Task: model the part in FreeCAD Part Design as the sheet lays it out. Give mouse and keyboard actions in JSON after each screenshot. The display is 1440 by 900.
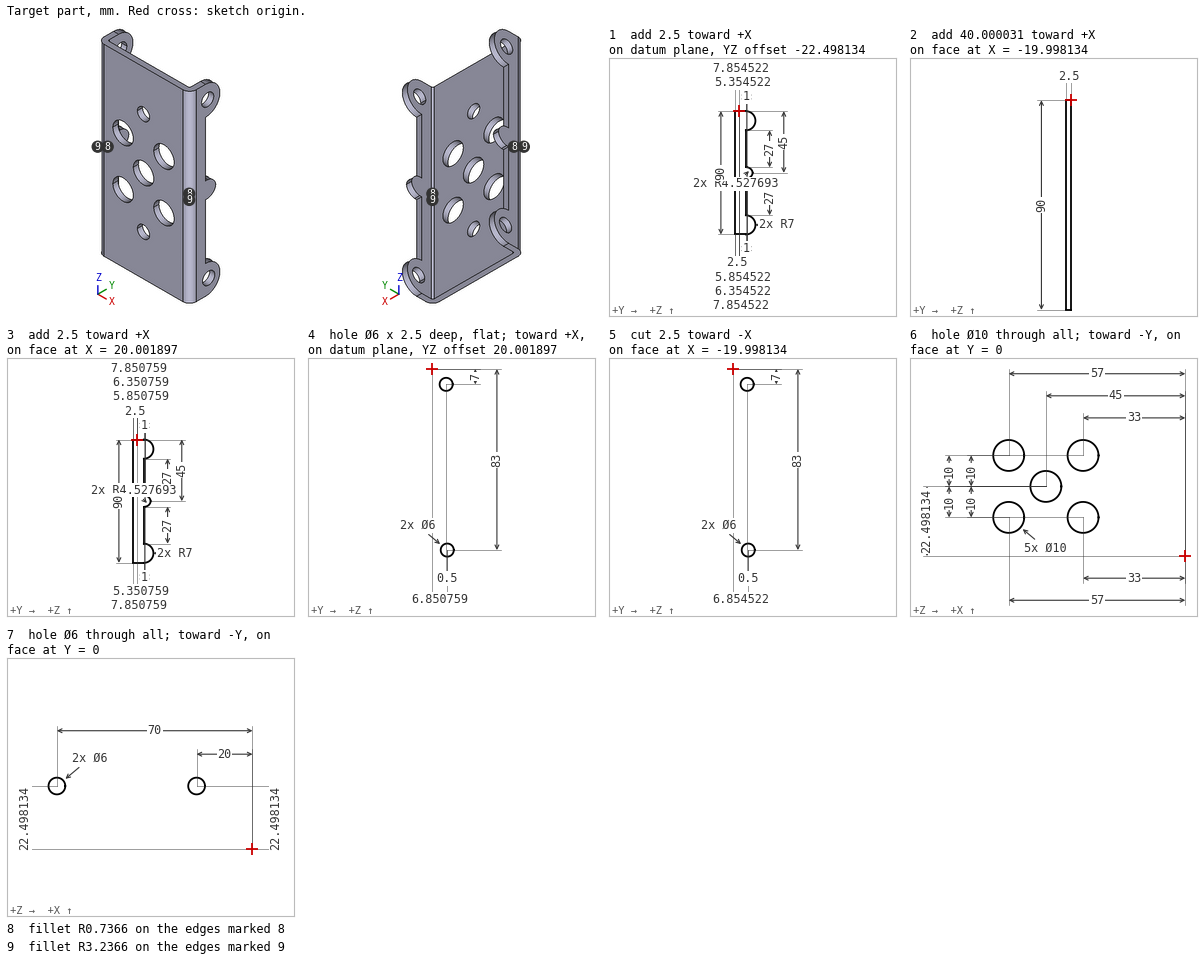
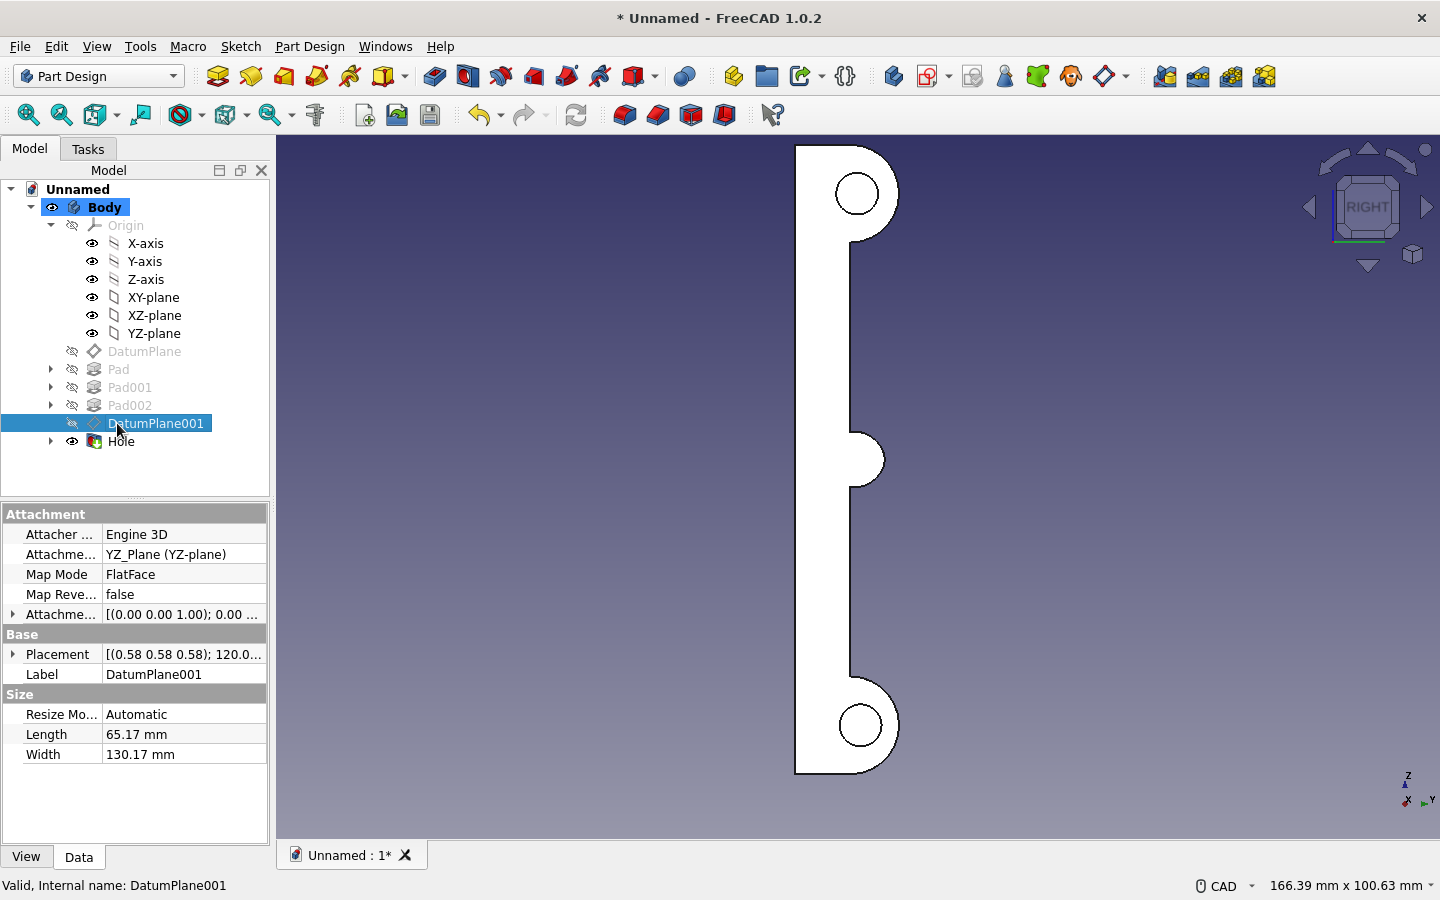
{"action": "left_click", "coordinate": [856, 728]}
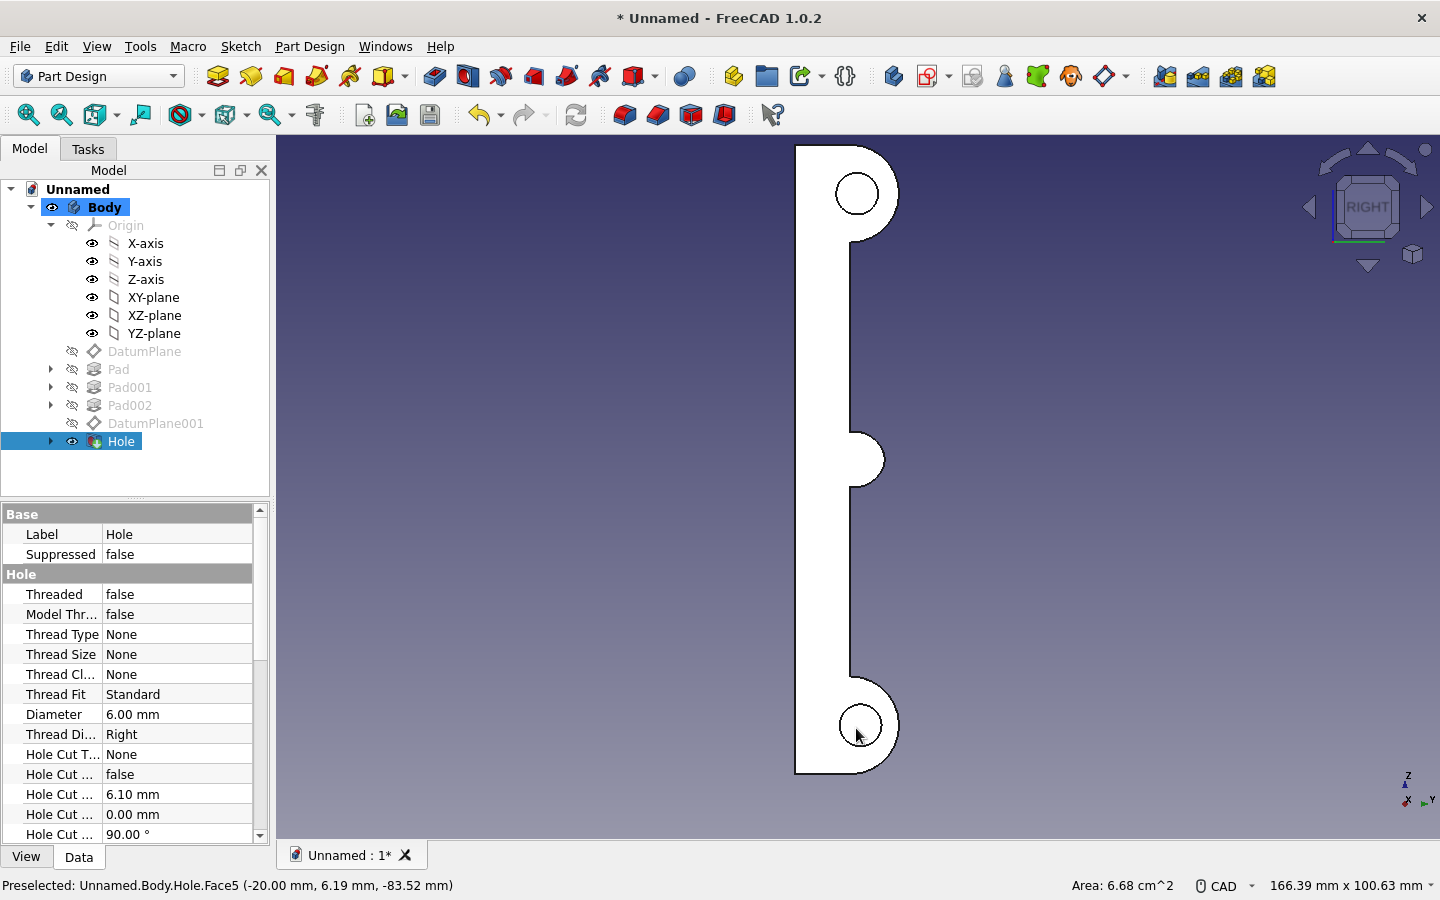
{"action": "left_click", "coordinate": [926, 76]}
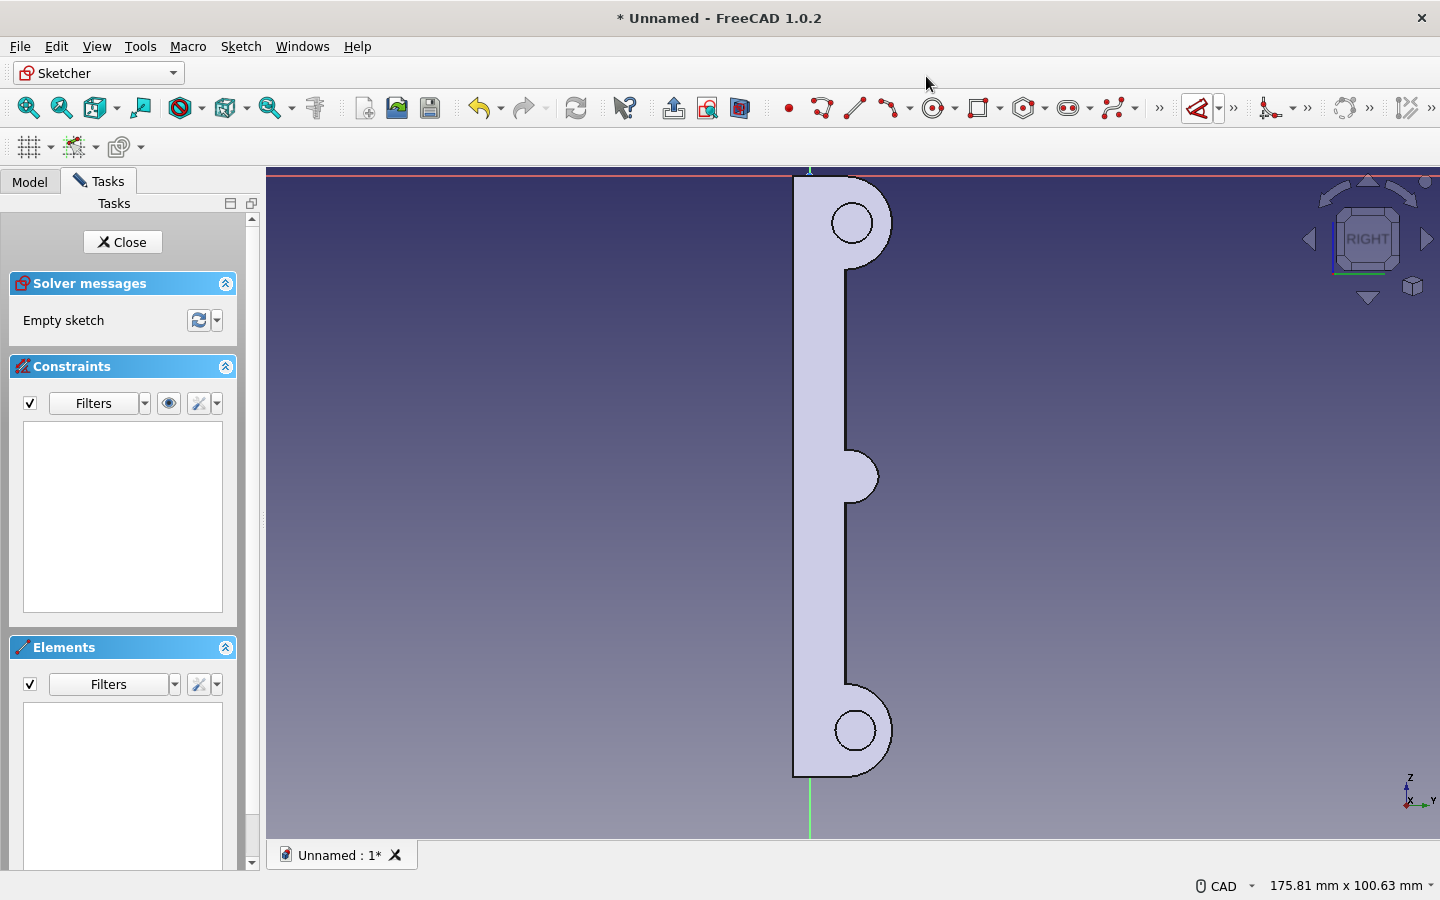
{"action": "key", "text": "q s"}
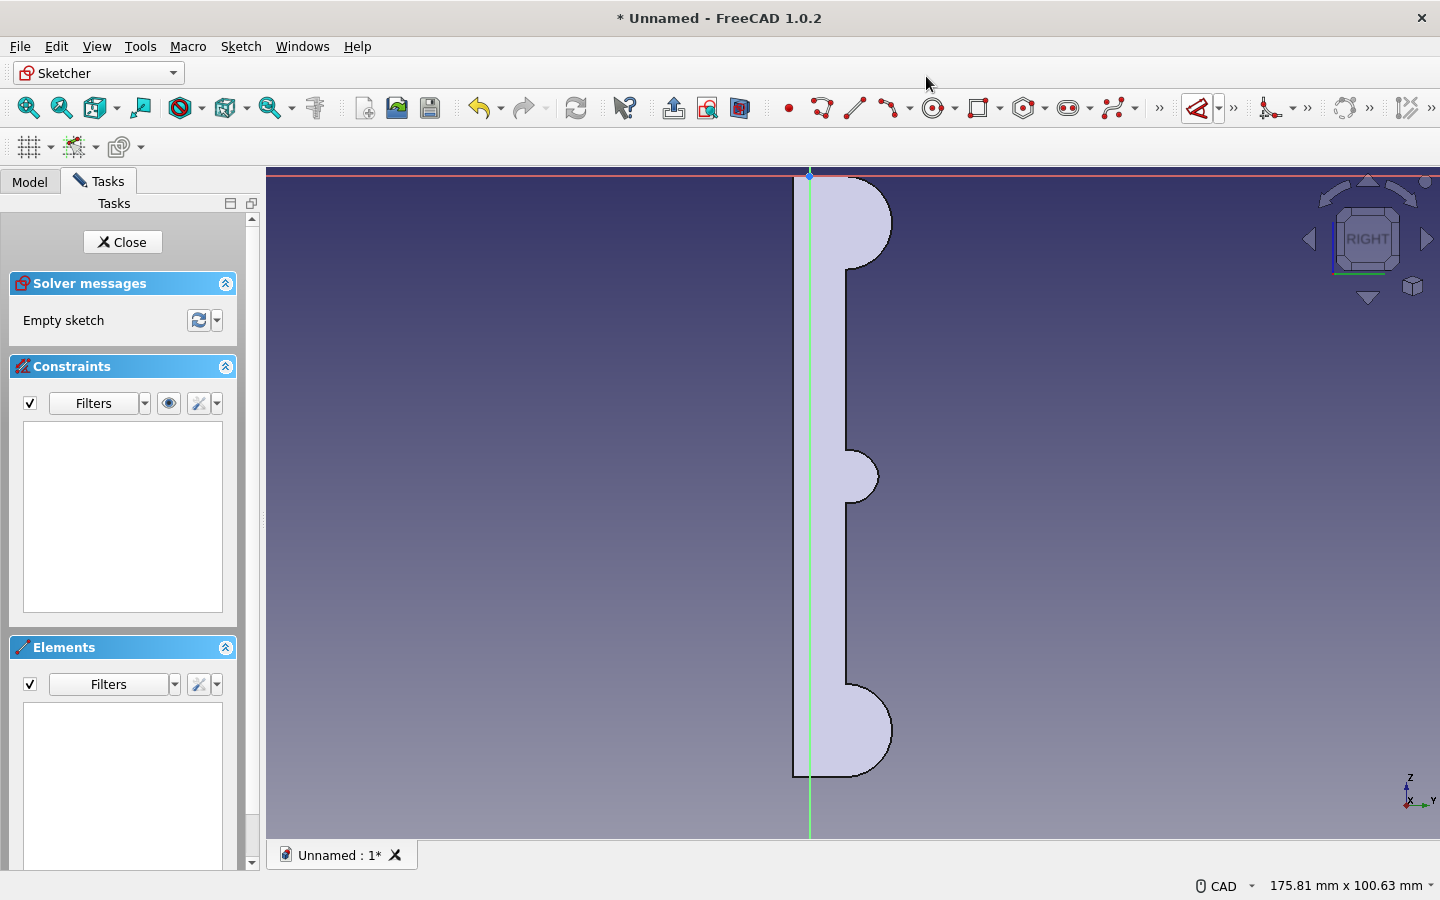
{"action": "scroll", "coordinate": [522, 682], "scroll_direction": "down", "scroll_amount": 1}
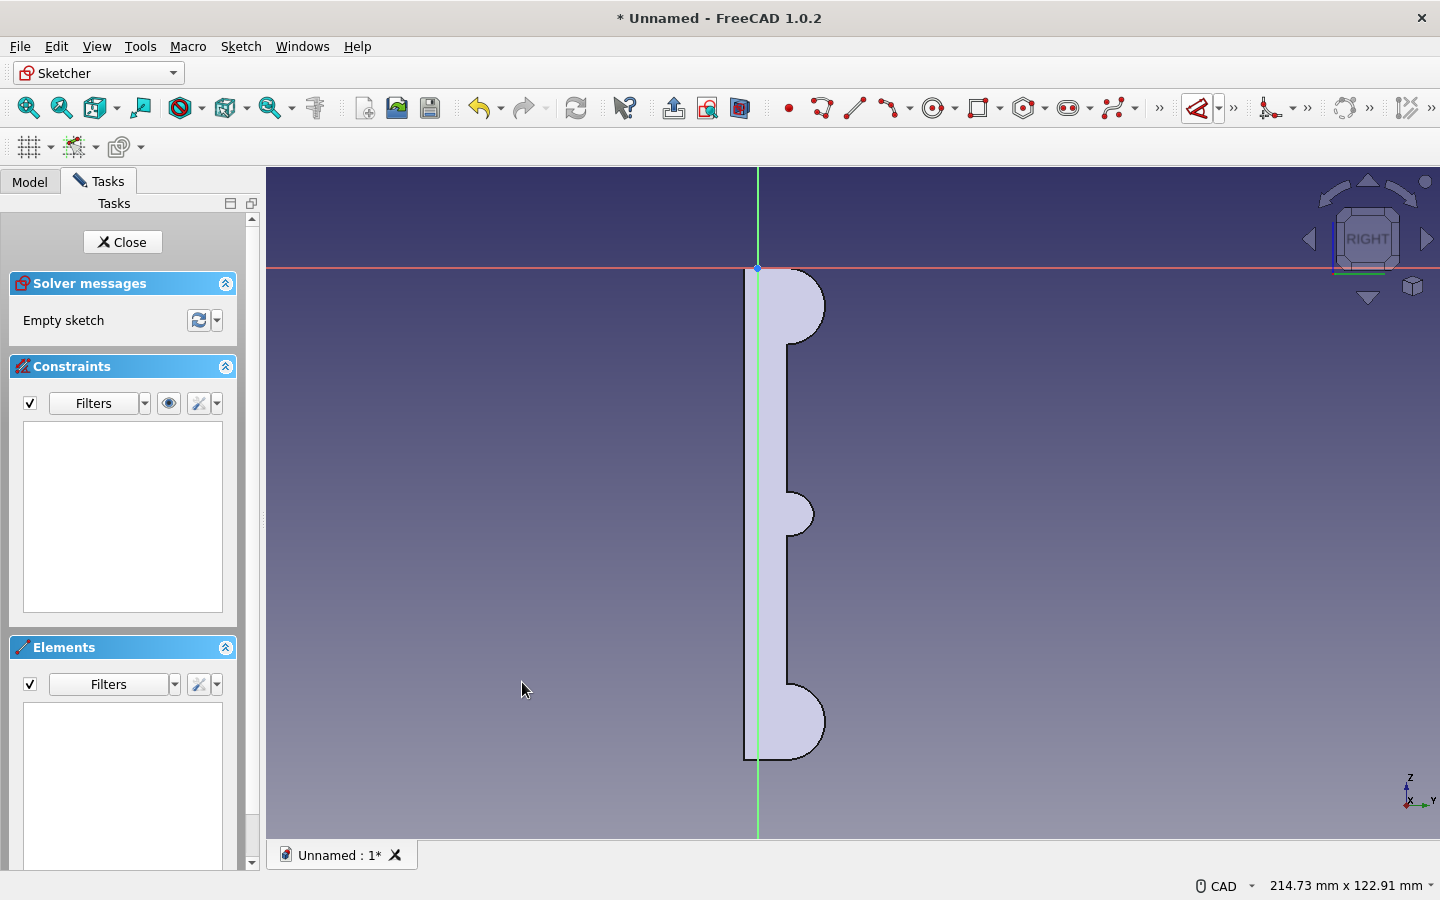
{"action": "left_click", "coordinate": [932, 108]}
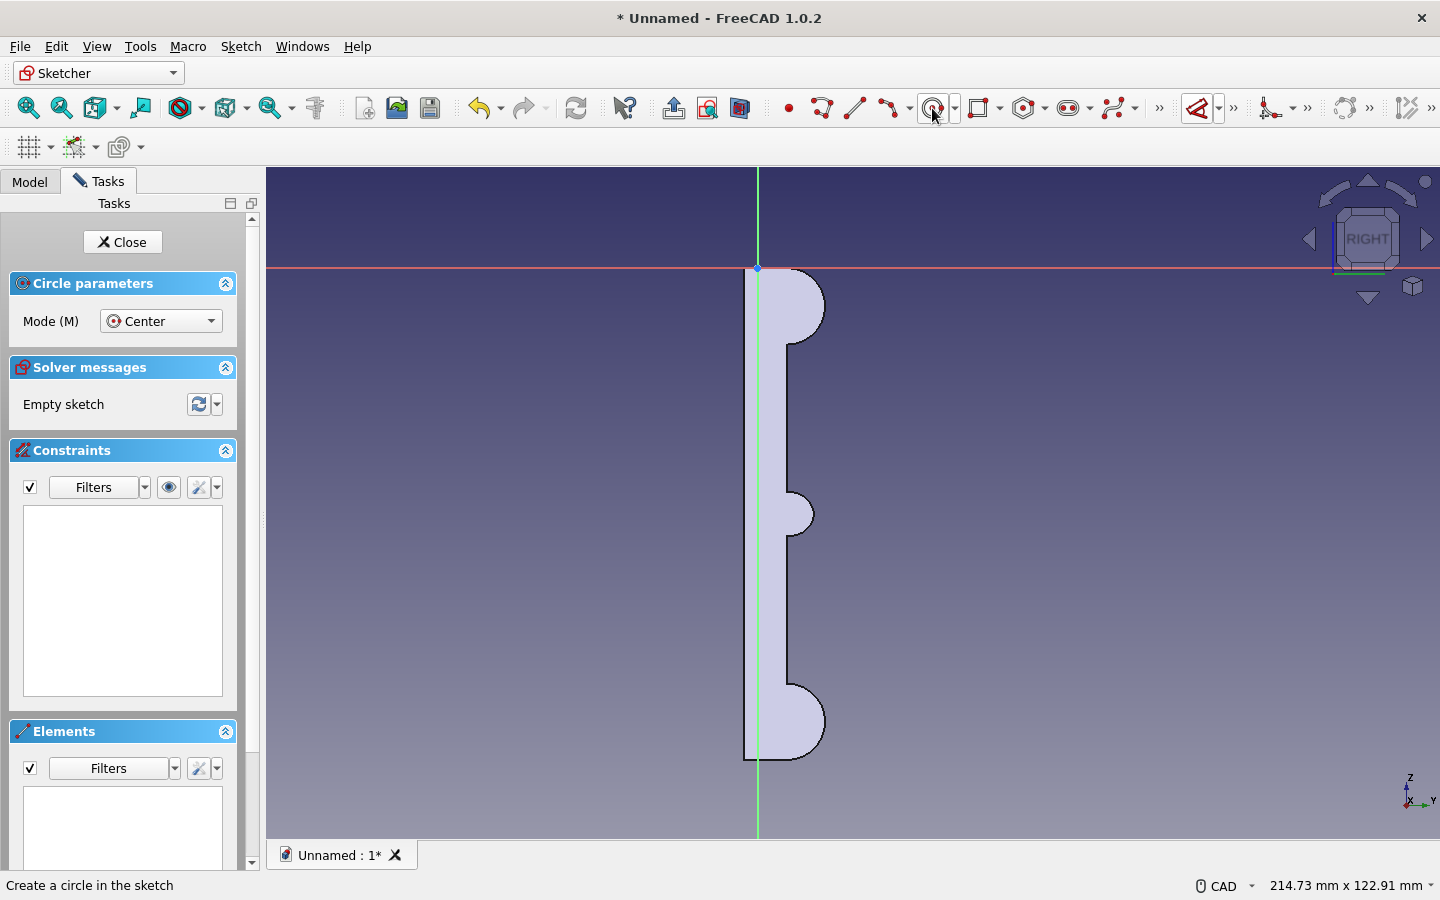
{"action": "scroll", "coordinate": [795, 722], "scroll_direction": "up", "scroll_amount": 2}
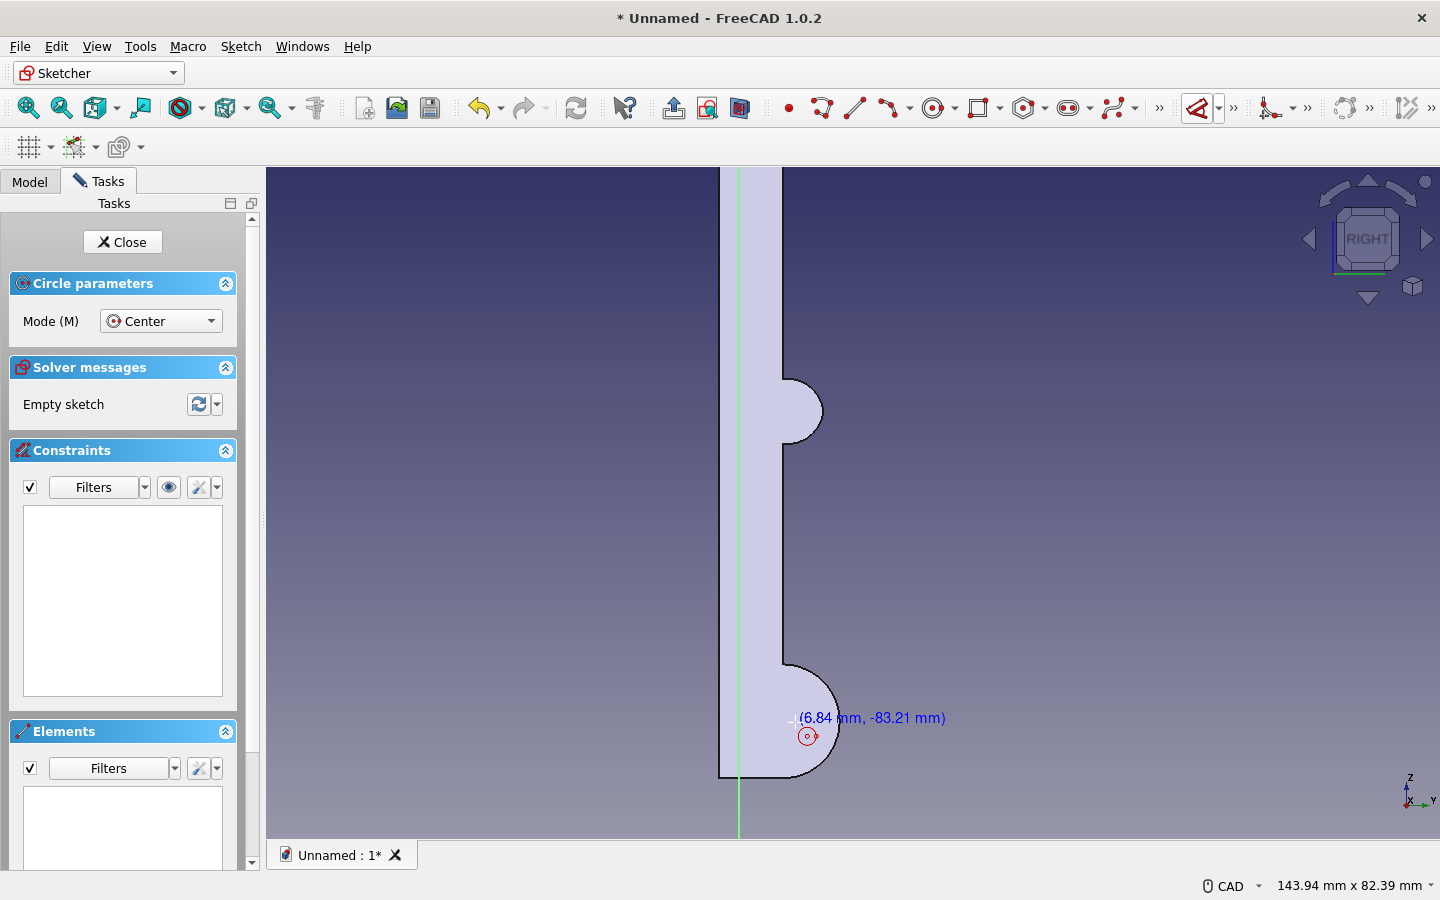
{"action": "left_click", "coordinate": [795, 721]}
{"action": "mouse_move", "coordinate": [812, 704]}